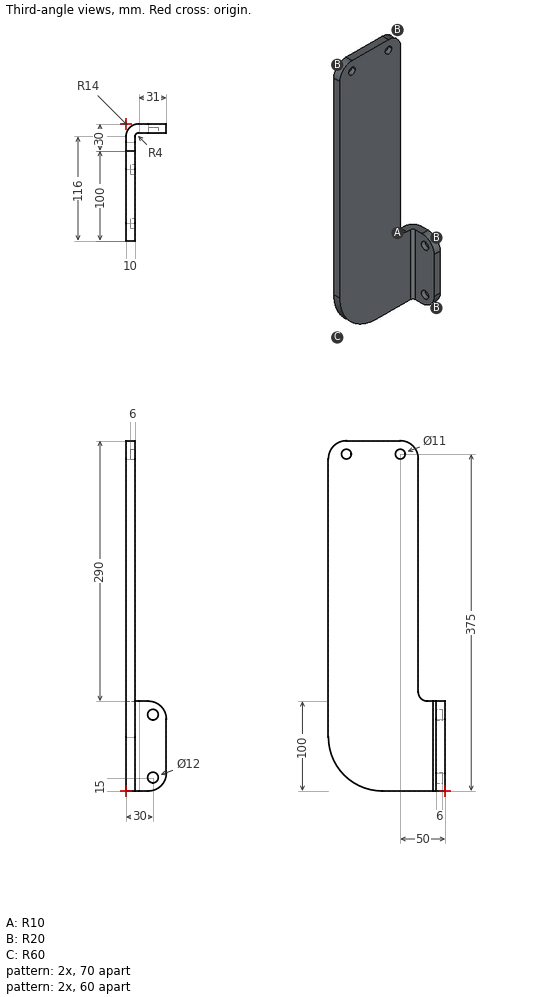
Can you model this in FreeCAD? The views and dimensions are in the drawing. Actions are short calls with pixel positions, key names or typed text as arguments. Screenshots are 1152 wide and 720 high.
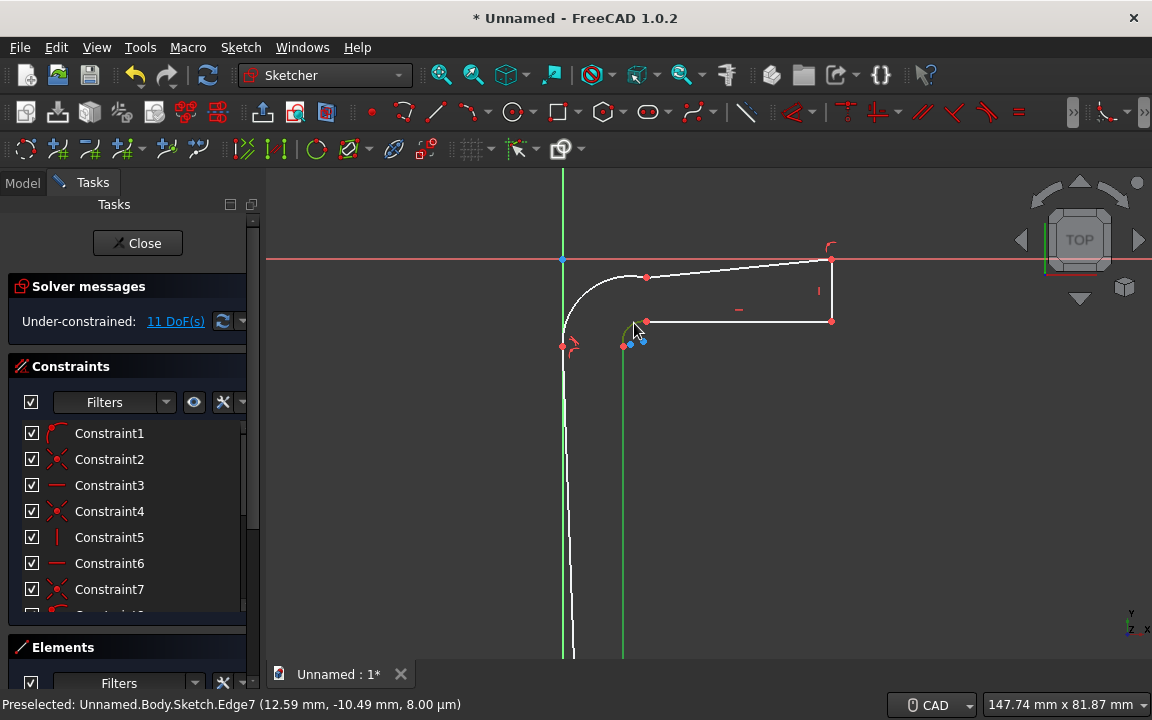
click(988, 112)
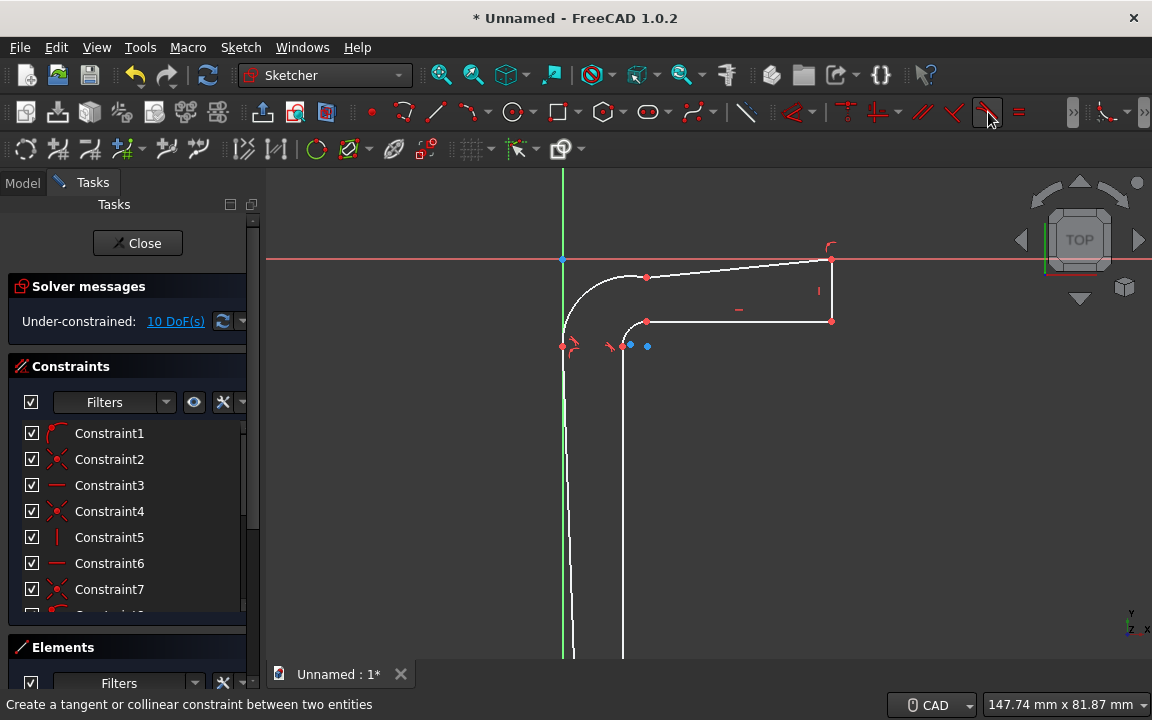
click(702, 322)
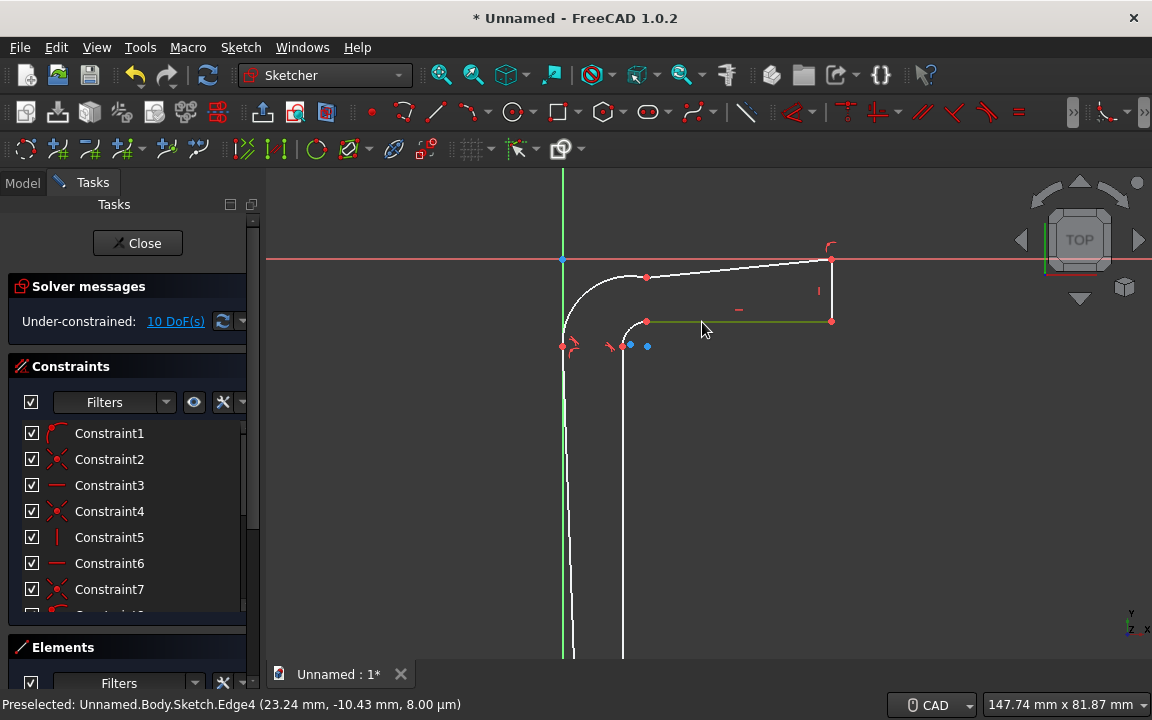
scroll(635, 325, up, 2)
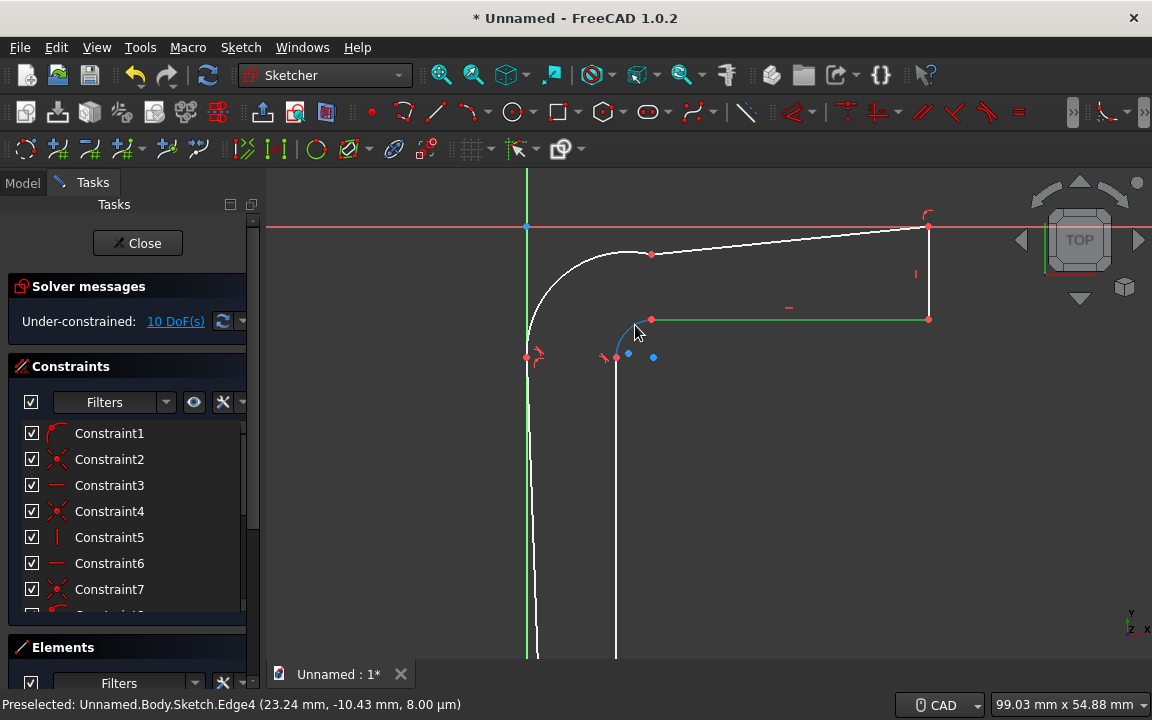
click(635, 325)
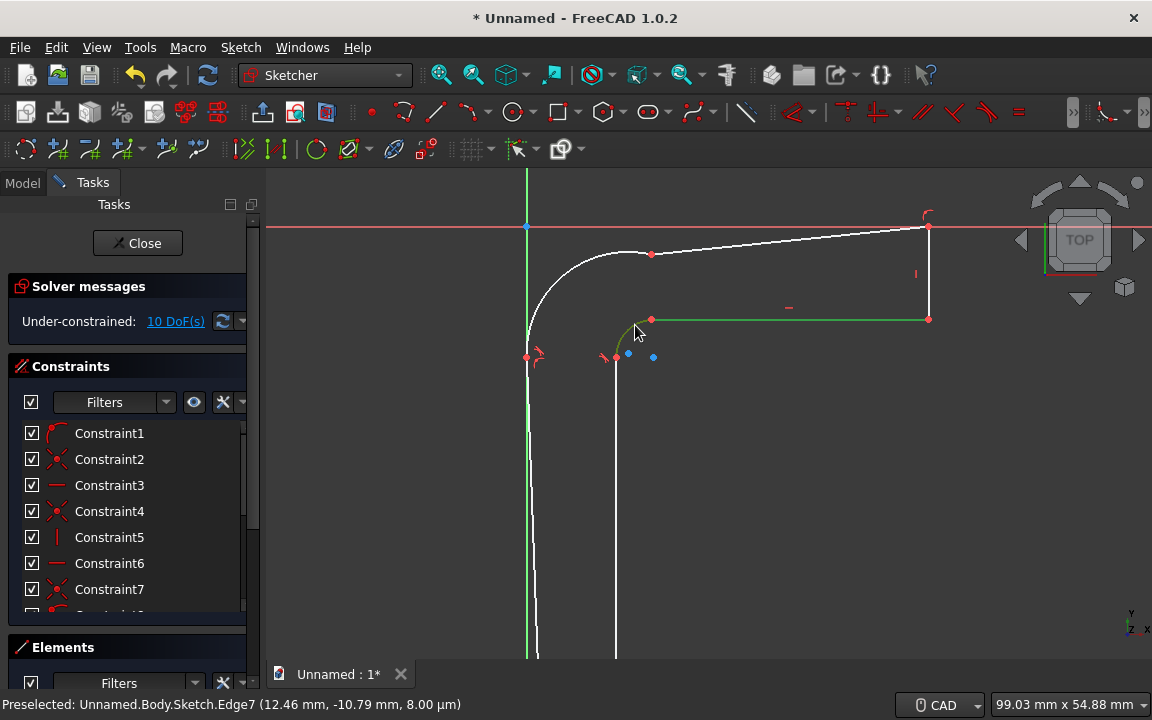
click(988, 112)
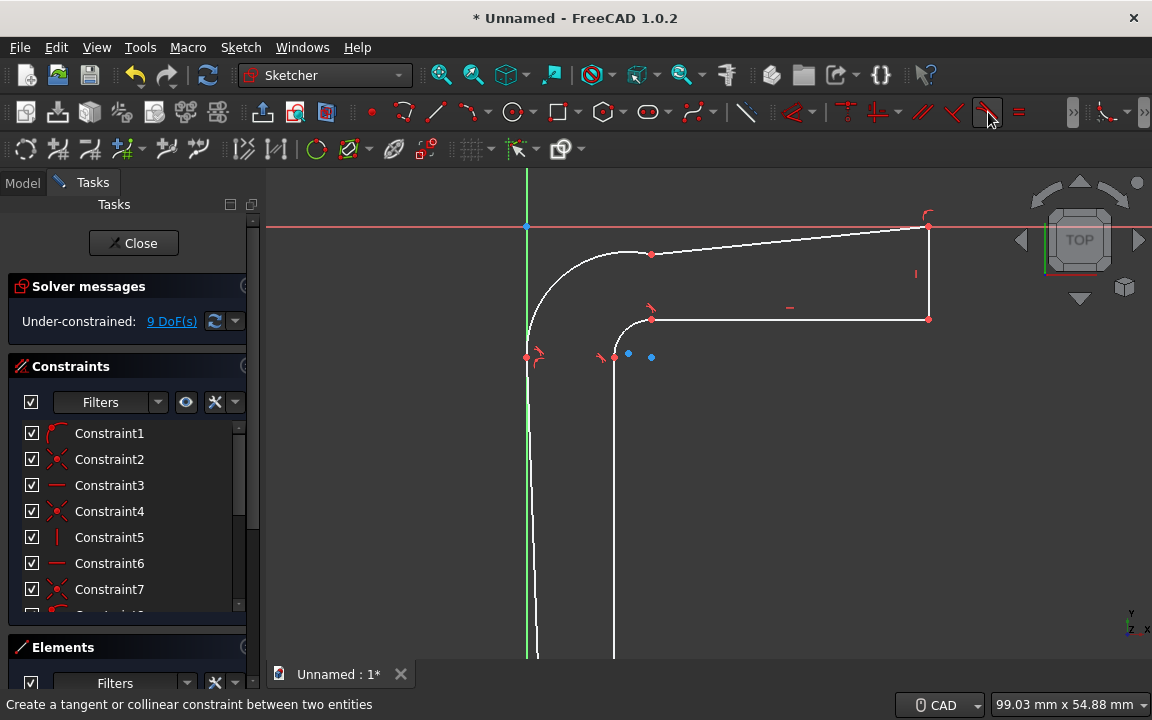
click(735, 246)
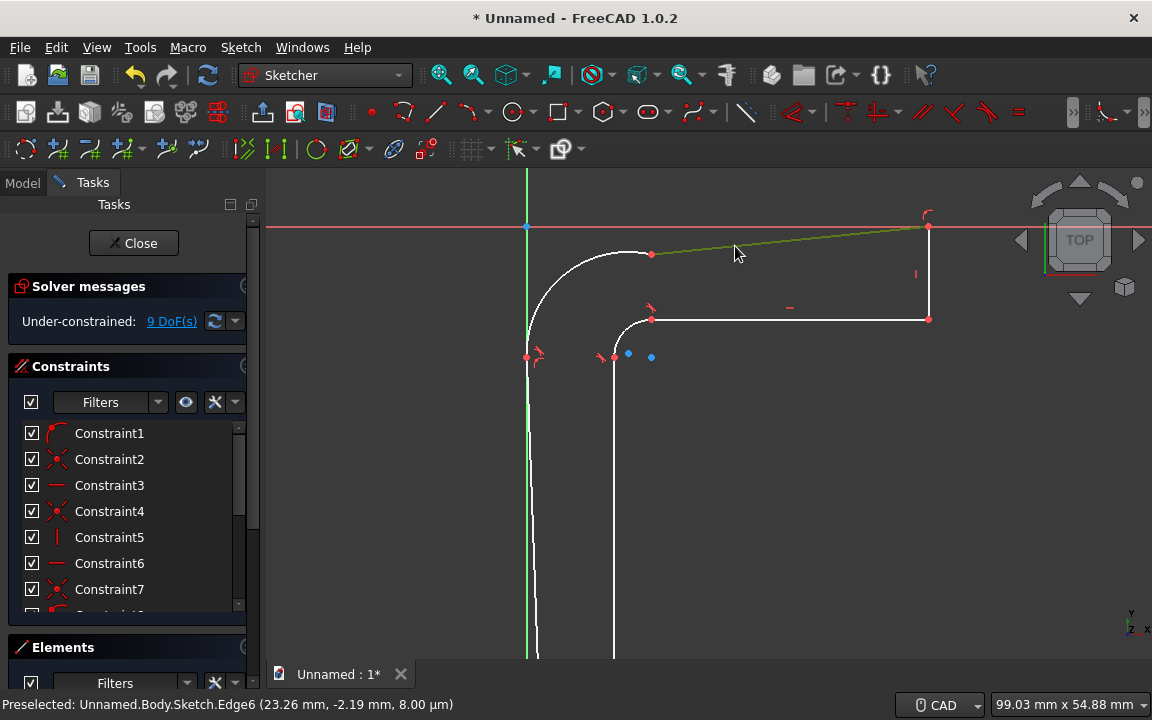
click(596, 257)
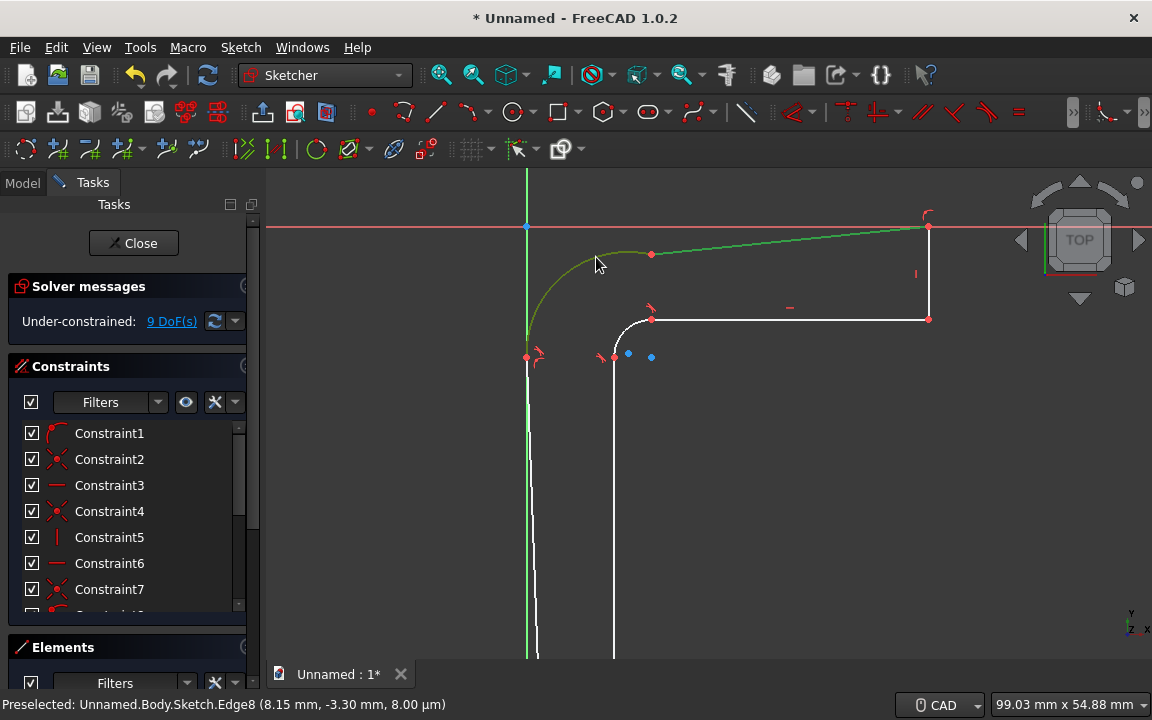
click(988, 112)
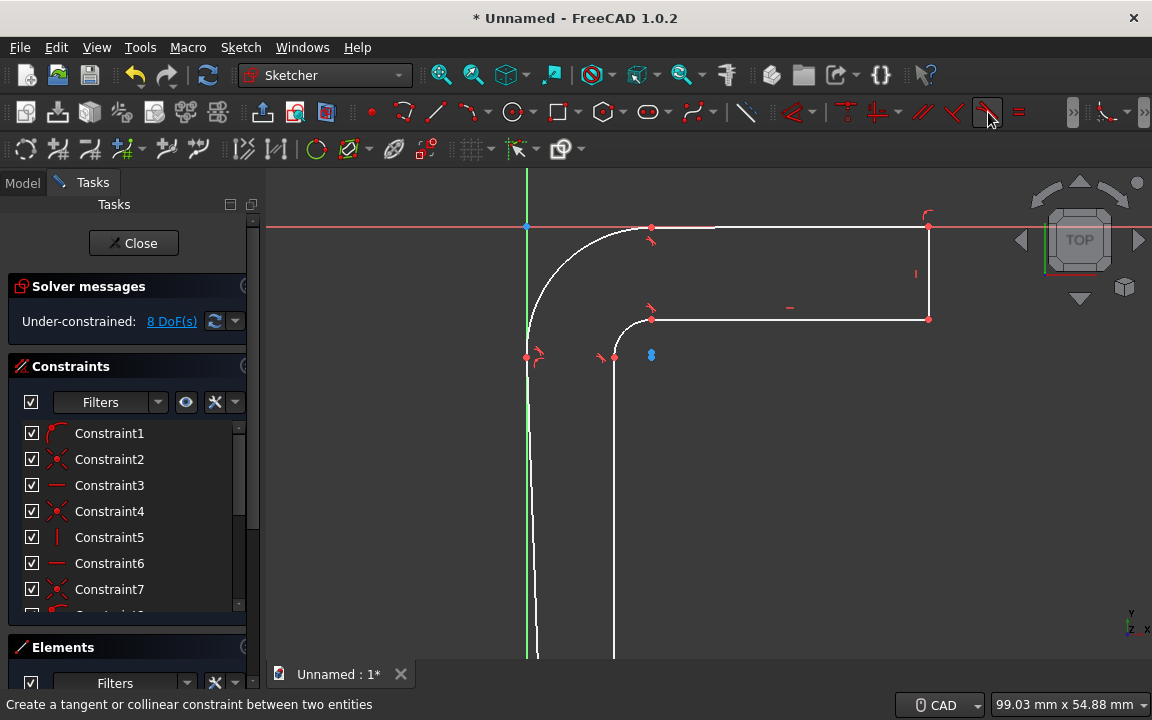
scroll(612, 284, down, 7)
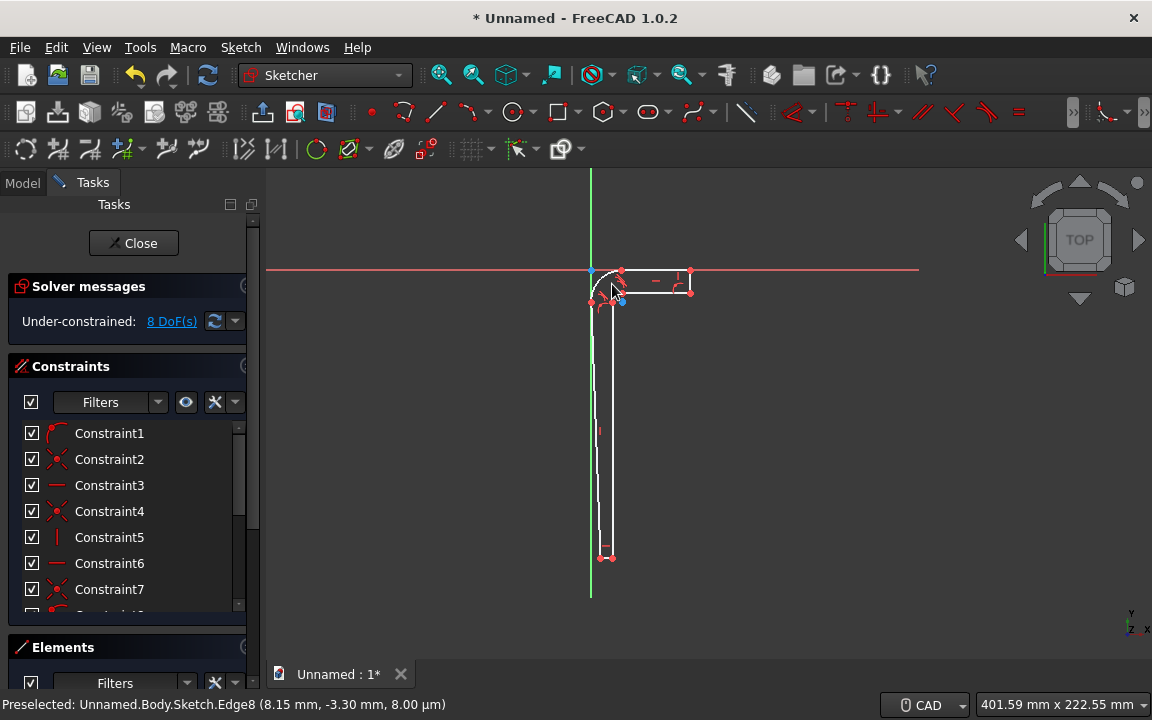
scroll(594, 379, up, 9)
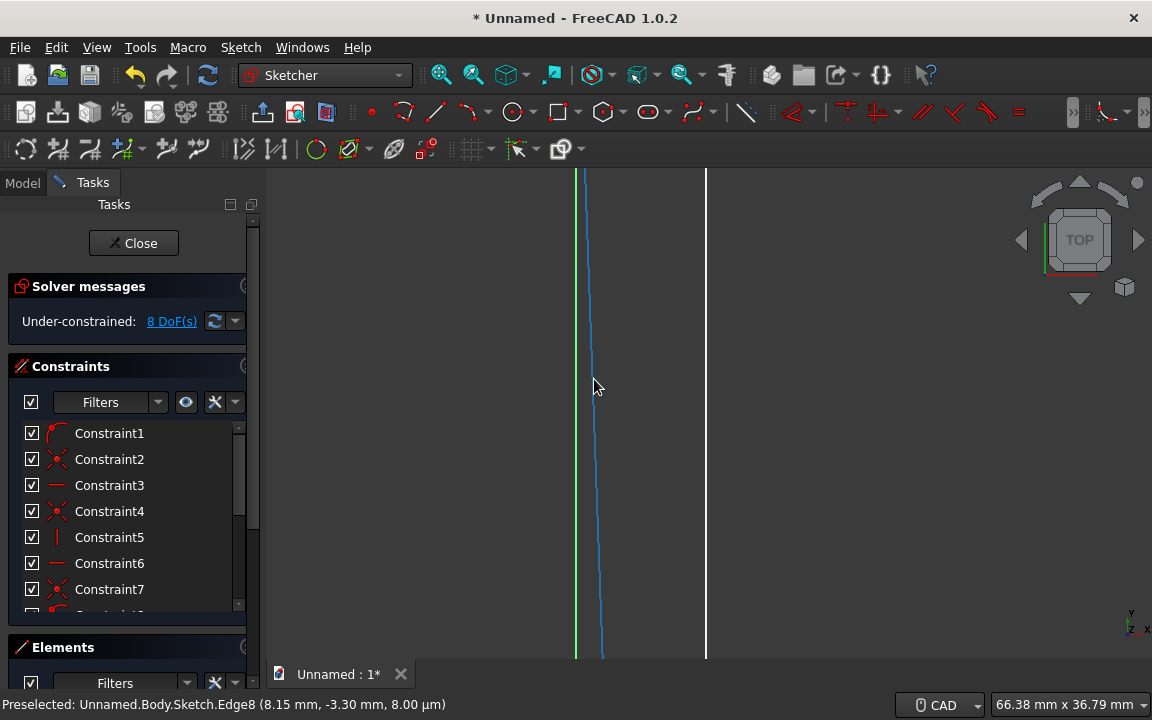
click(592, 377)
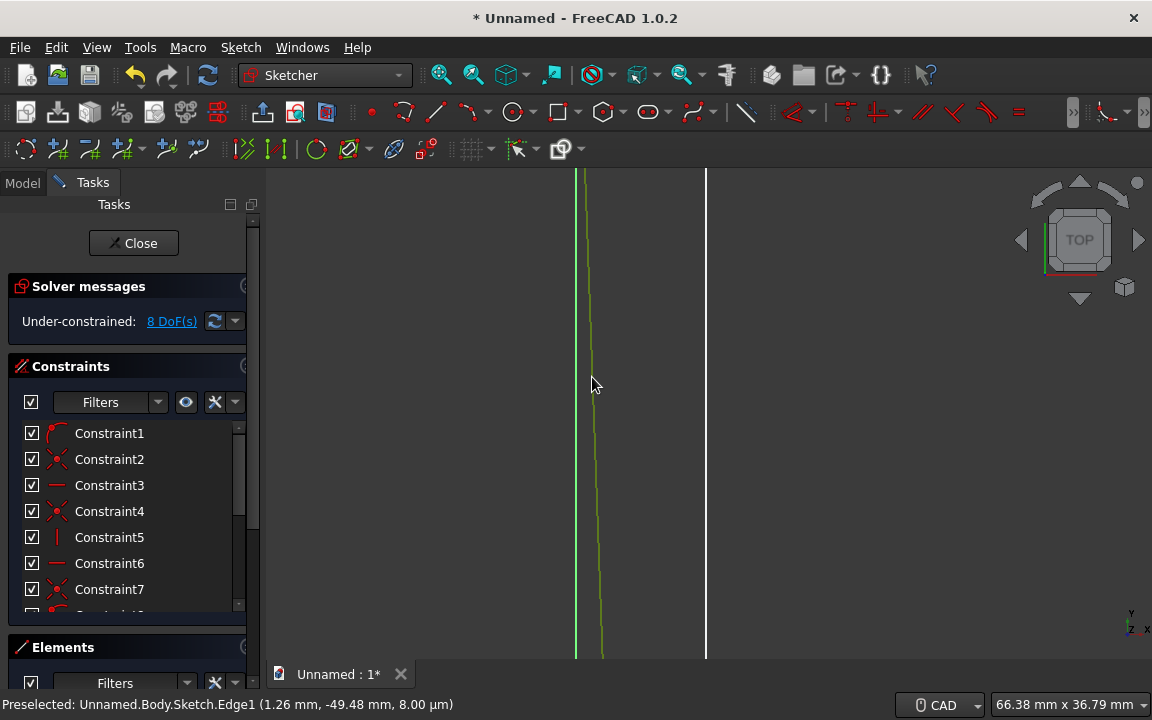
key(v)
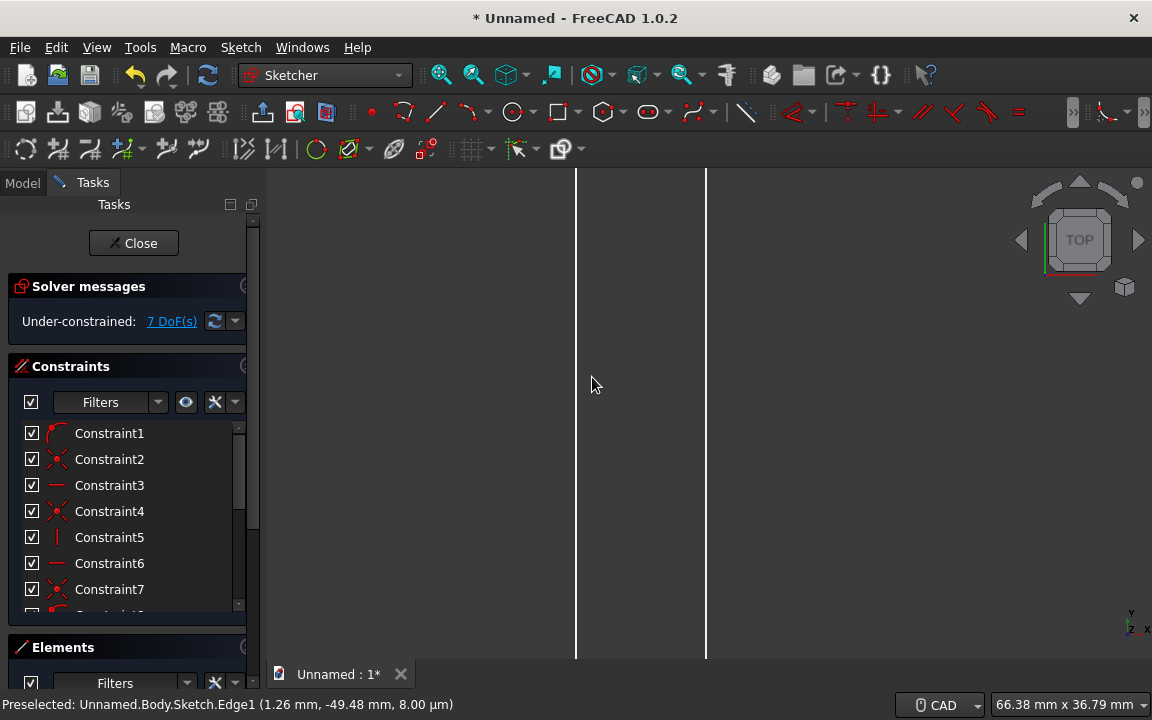
scroll(594, 380, down, 9)